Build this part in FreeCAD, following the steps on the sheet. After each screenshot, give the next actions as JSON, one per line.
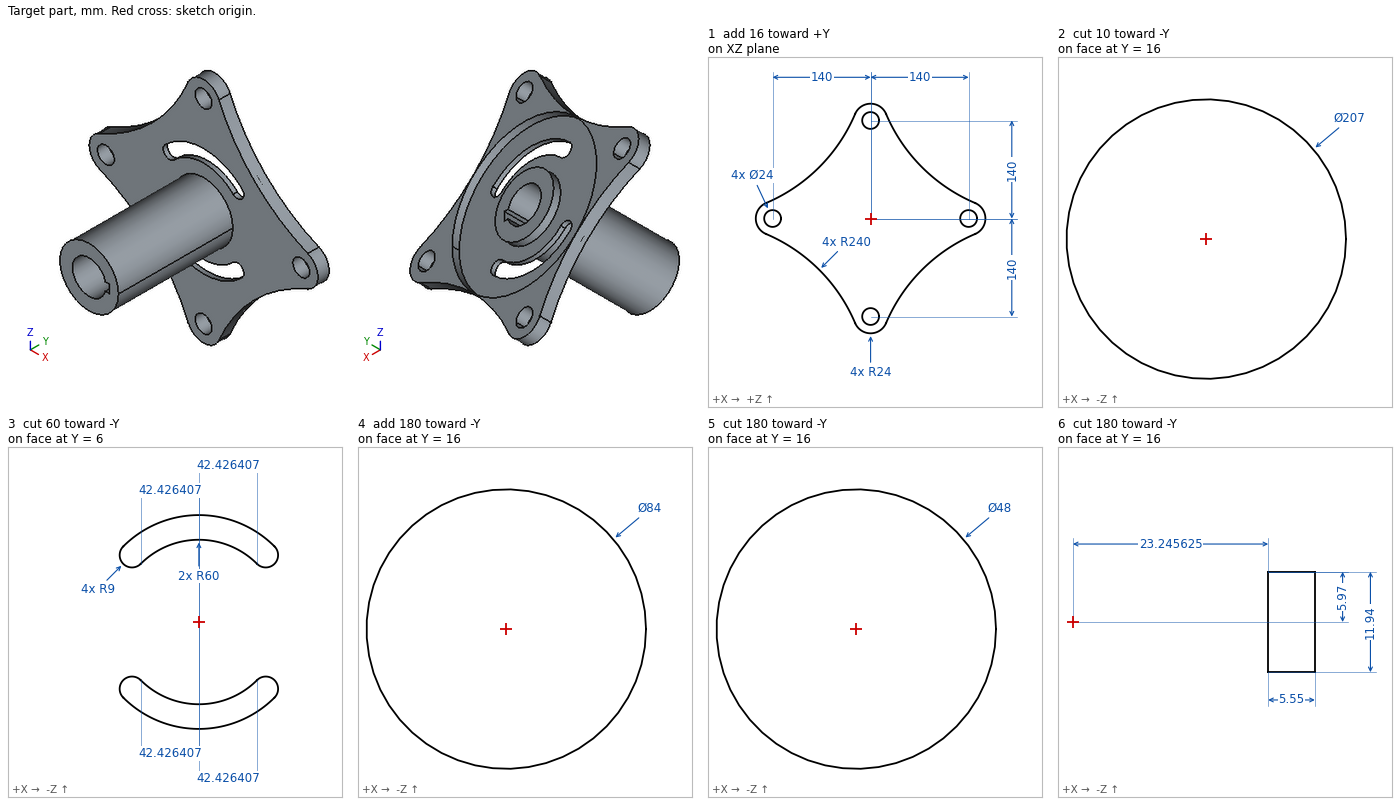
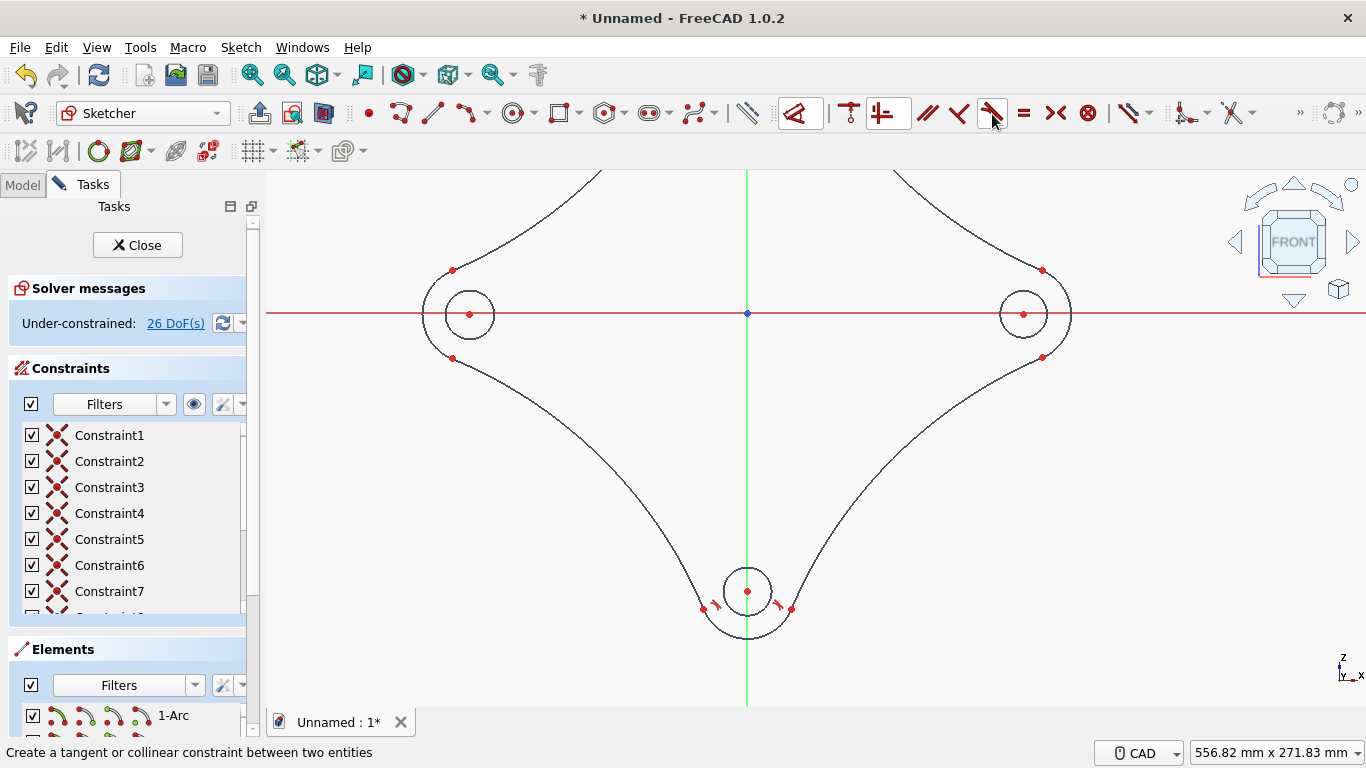
{"action": "left_click", "coordinate": [650, 515]}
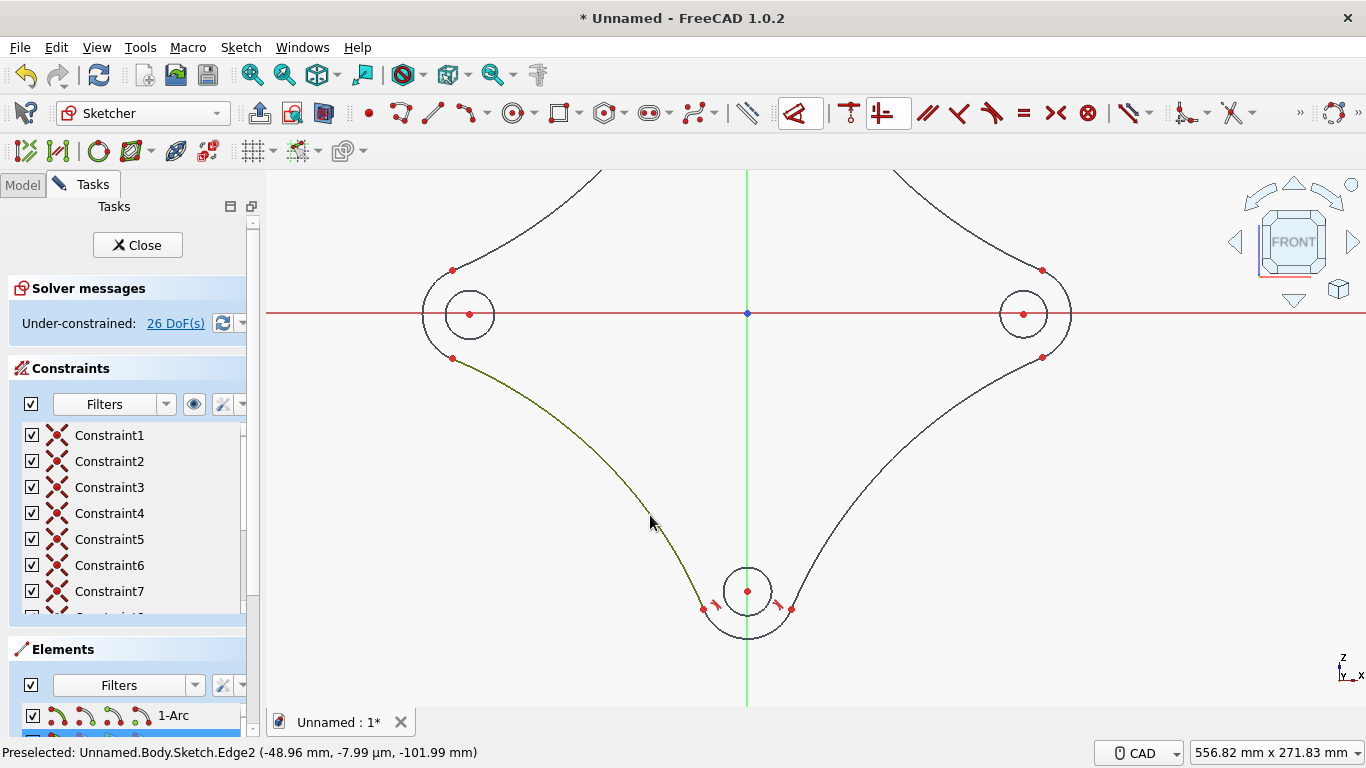
{"action": "left_click", "coordinate": [428, 293]}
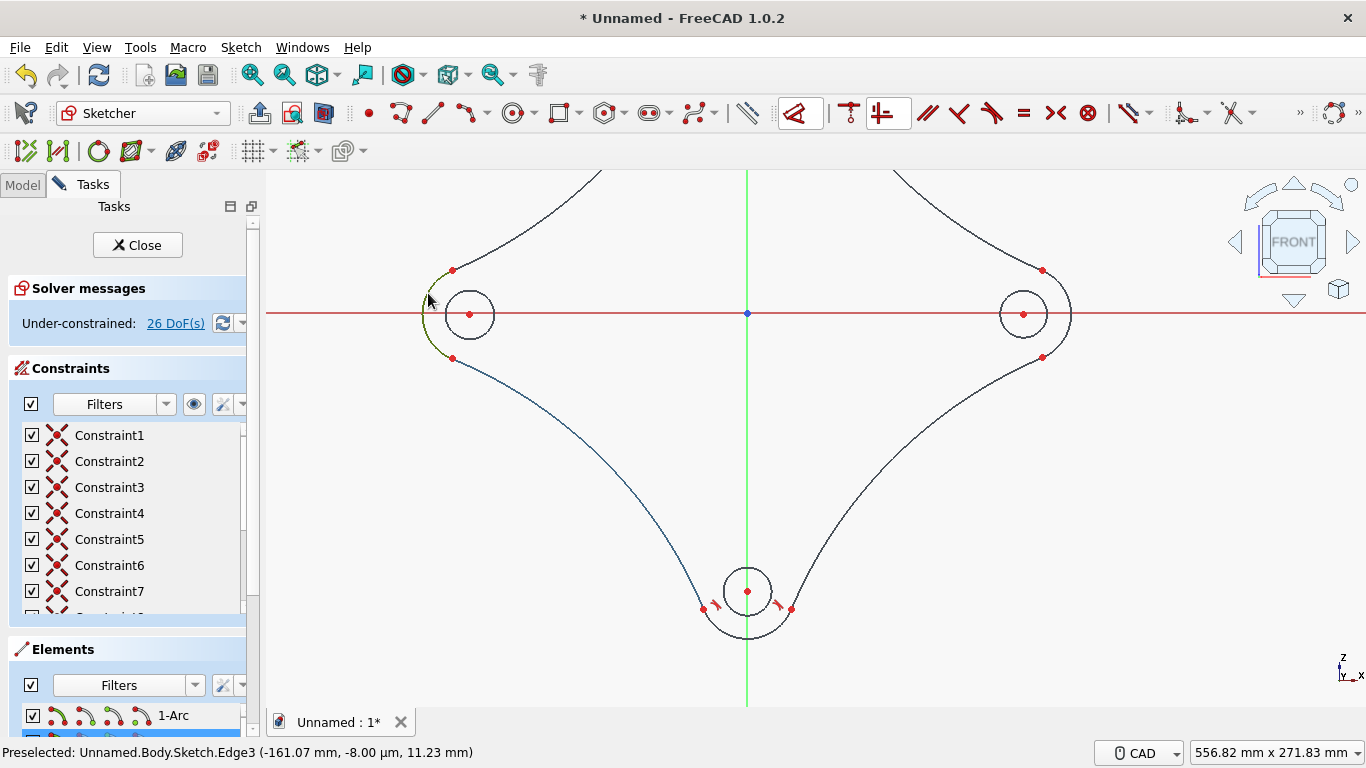
{"action": "left_click", "coordinate": [992, 114]}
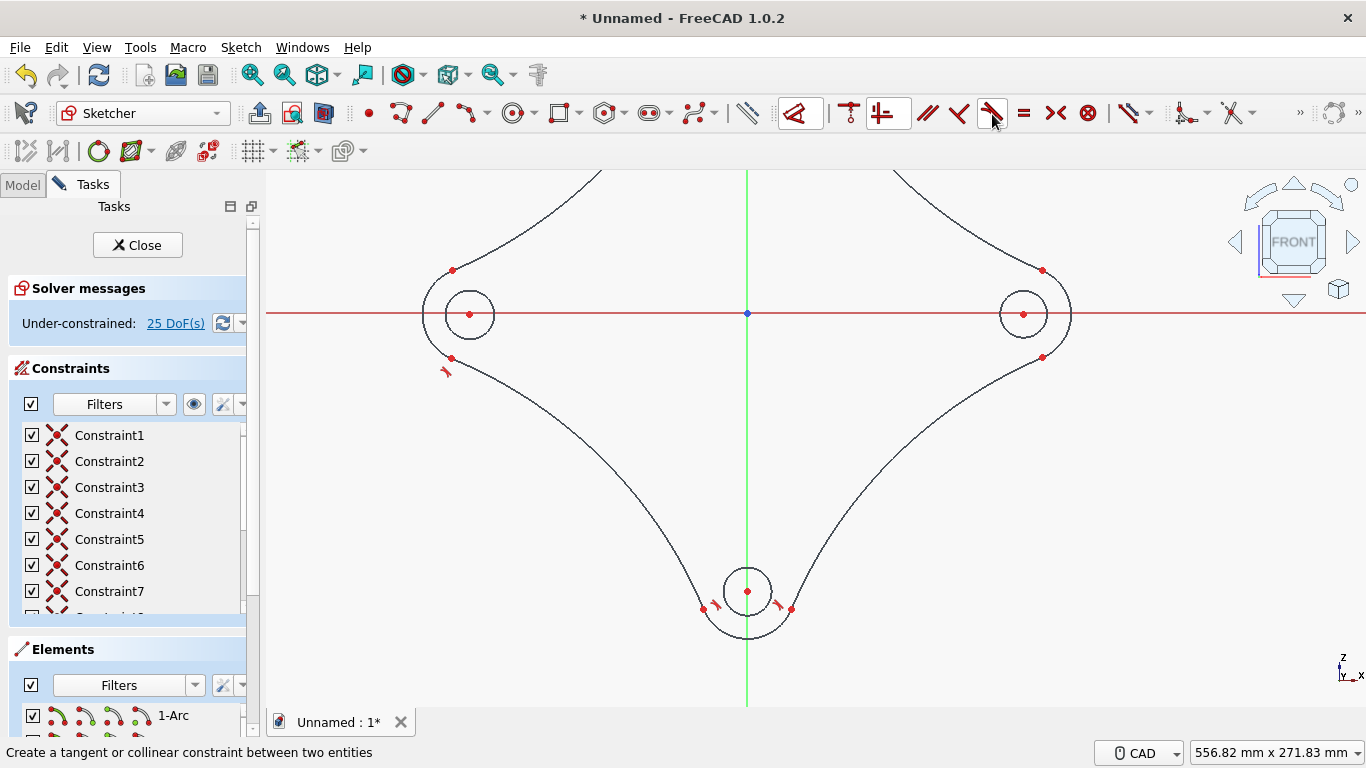
{"action": "left_click", "coordinate": [428, 293]}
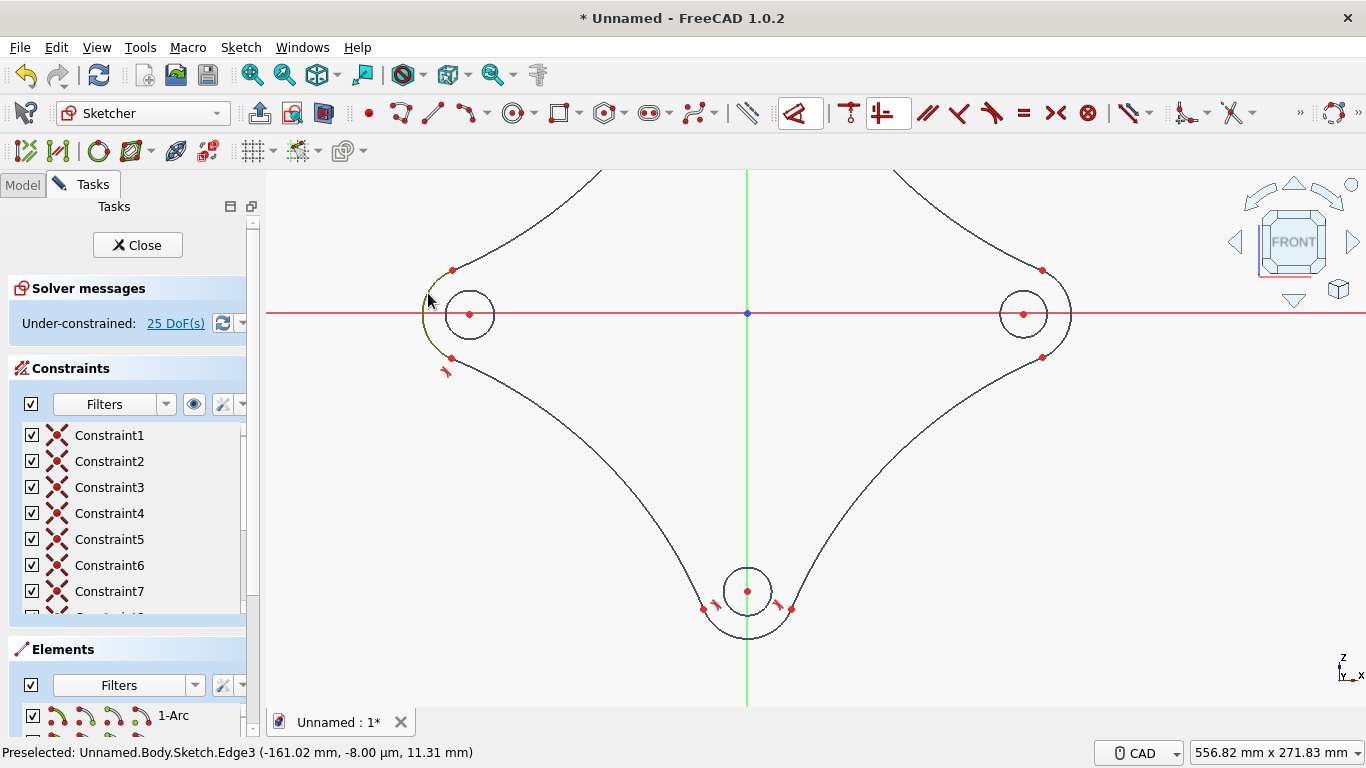
{"action": "left_click", "coordinate": [547, 217]}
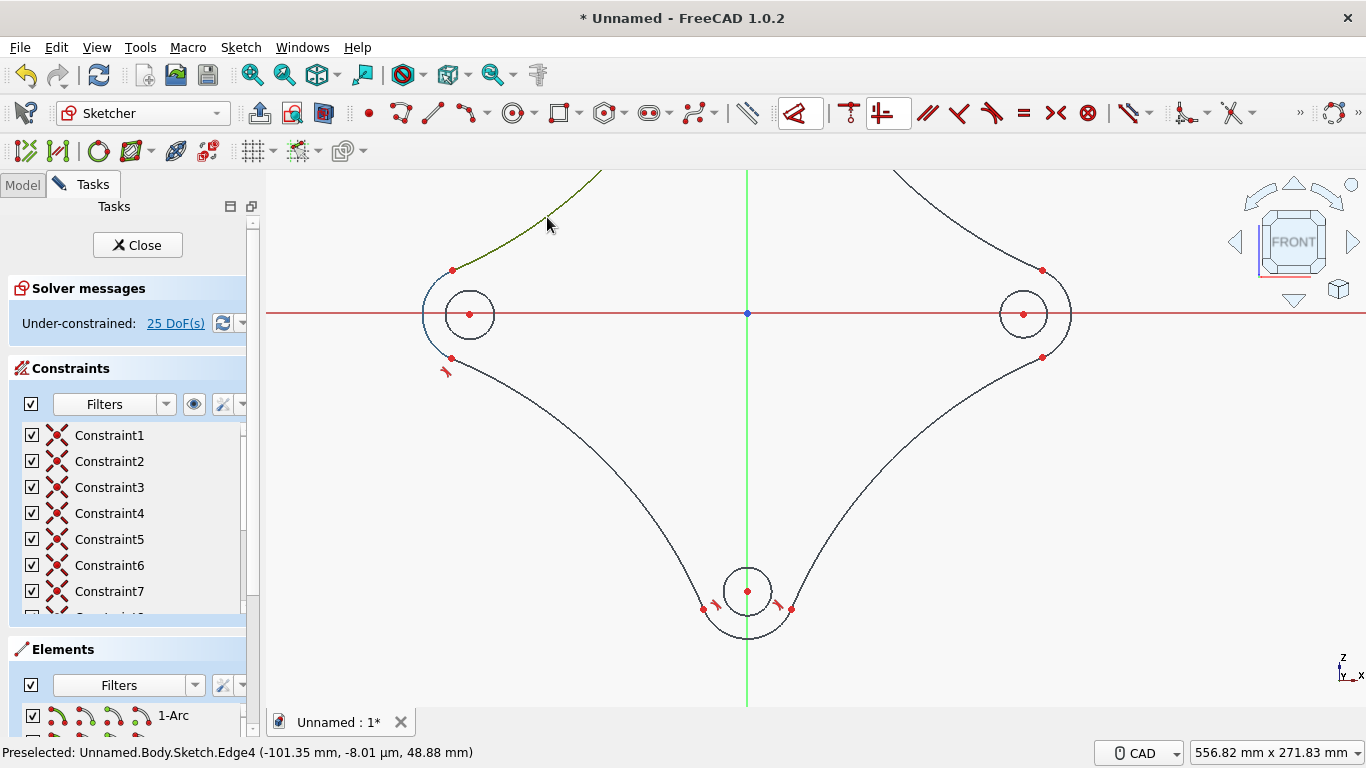
{"action": "left_click", "coordinate": [992, 114]}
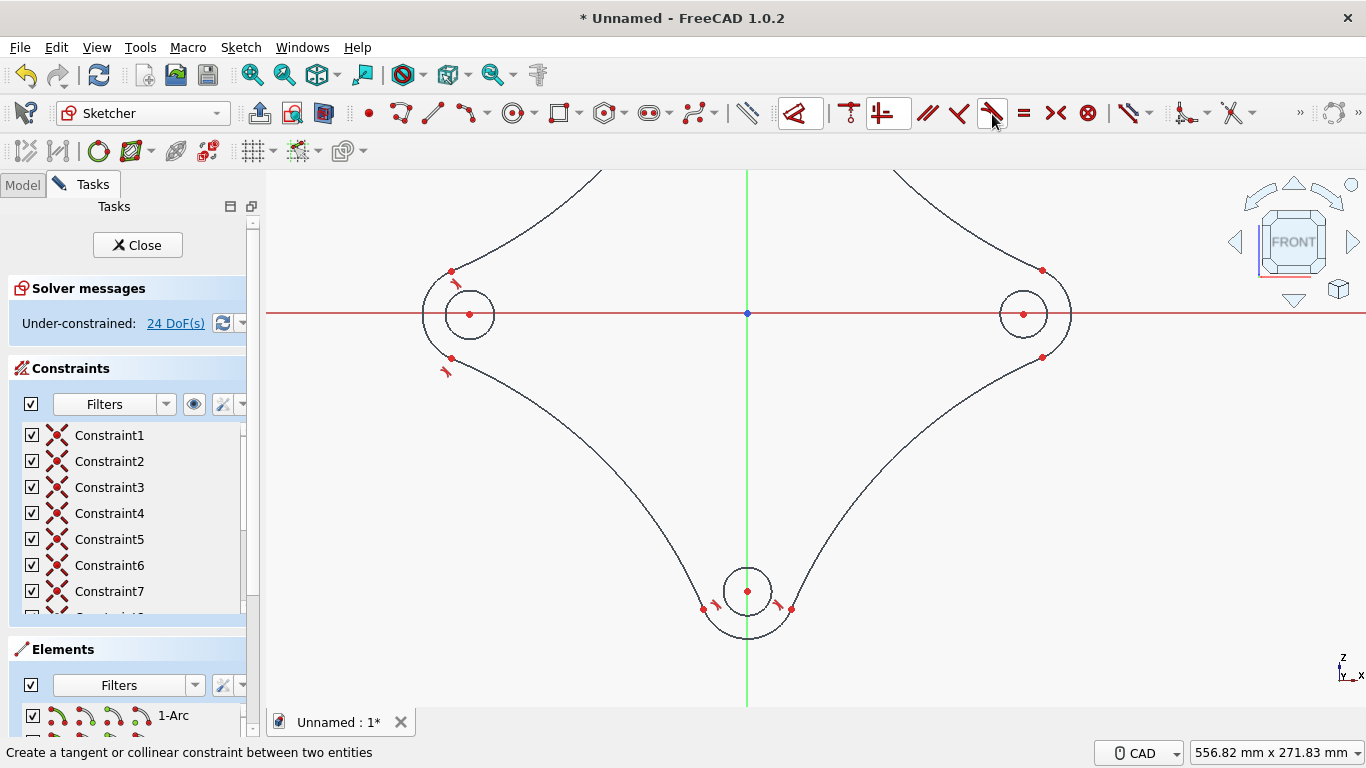
{"action": "left_click", "coordinate": [546, 217]}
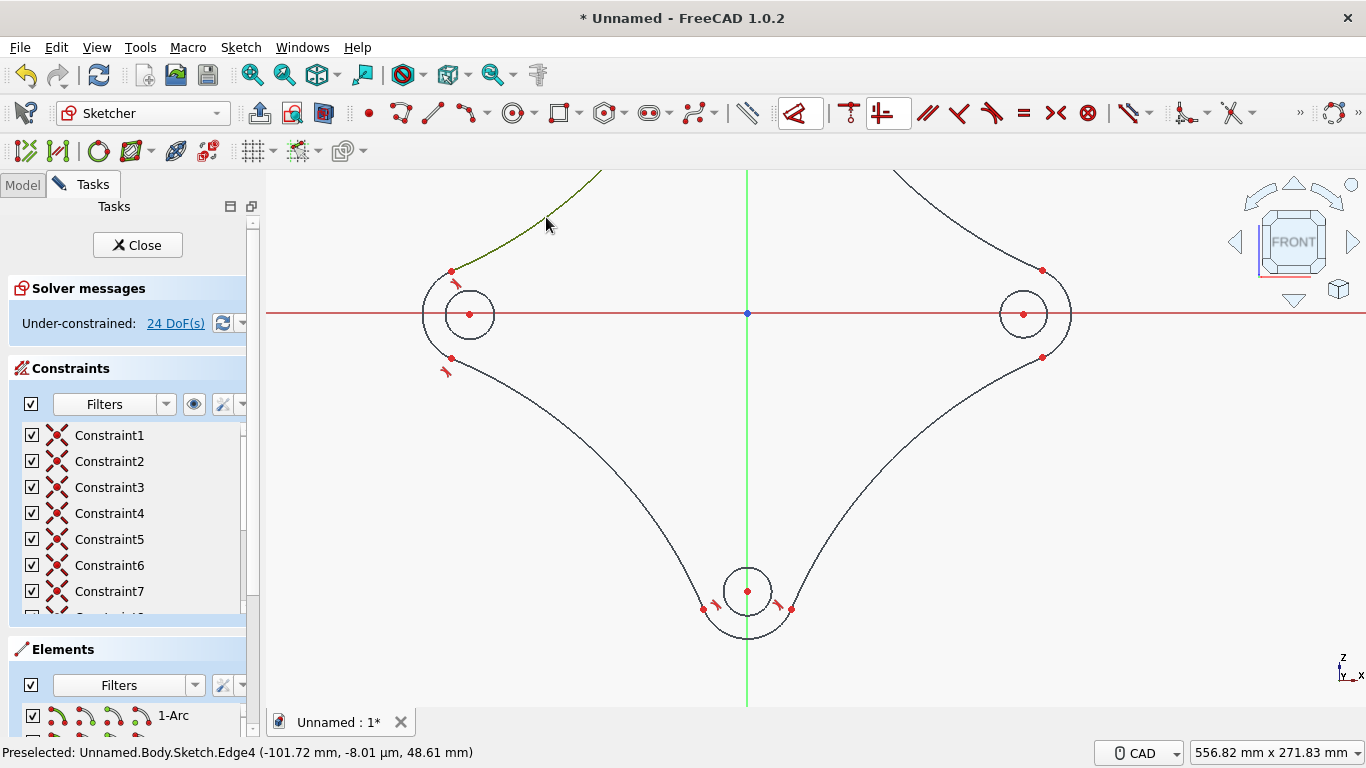
{"action": "scroll", "coordinate": [748, 591], "scroll_direction": "down", "scroll_amount": 3}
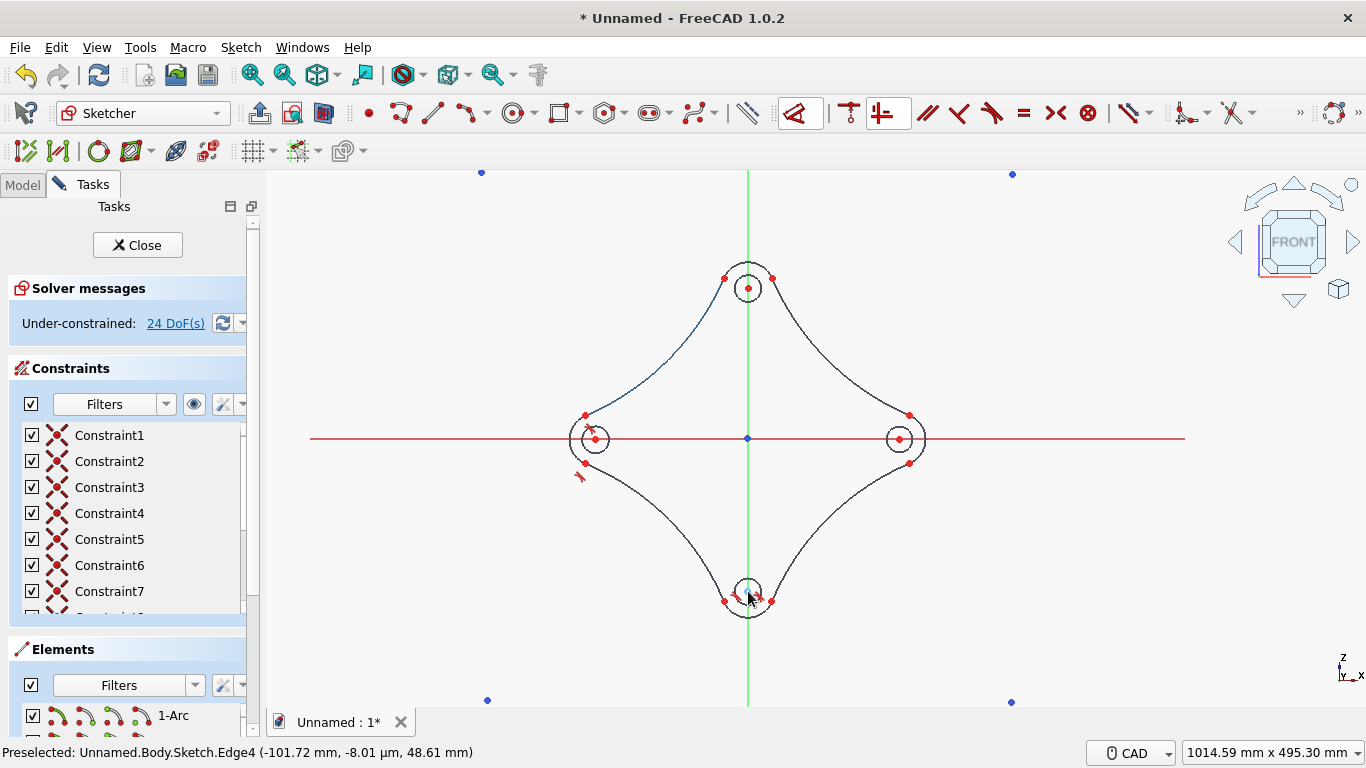
{"action": "left_click", "coordinate": [760, 265]}